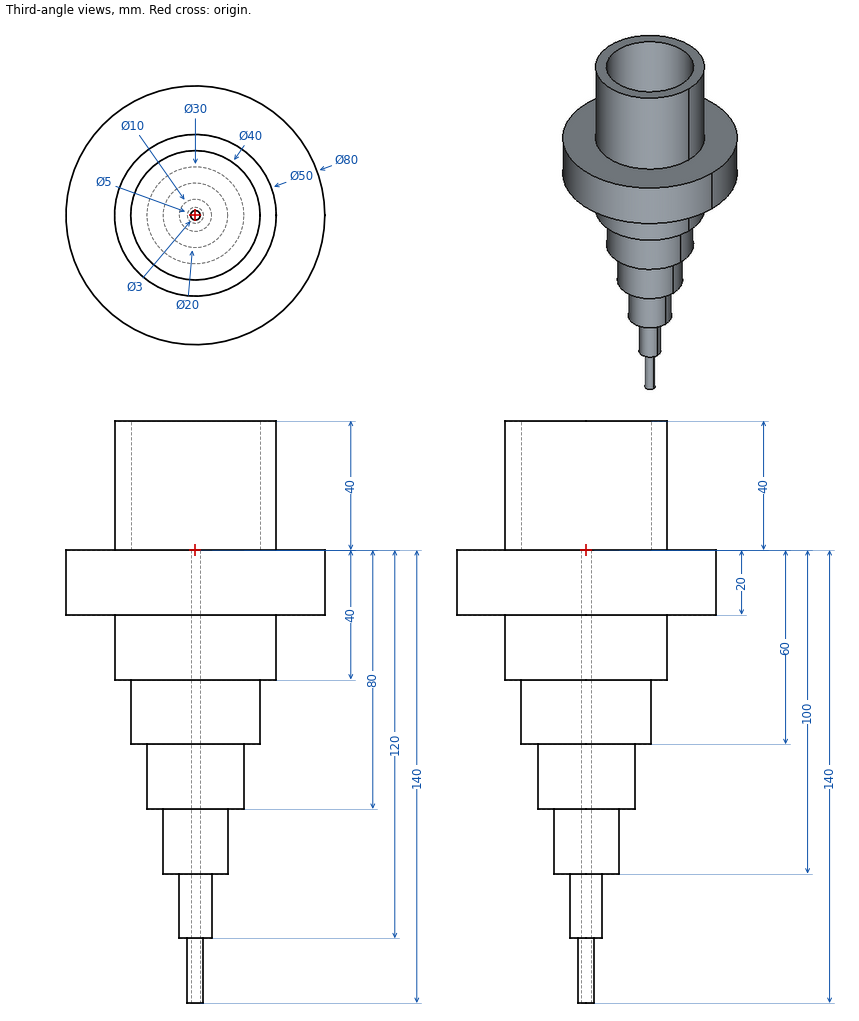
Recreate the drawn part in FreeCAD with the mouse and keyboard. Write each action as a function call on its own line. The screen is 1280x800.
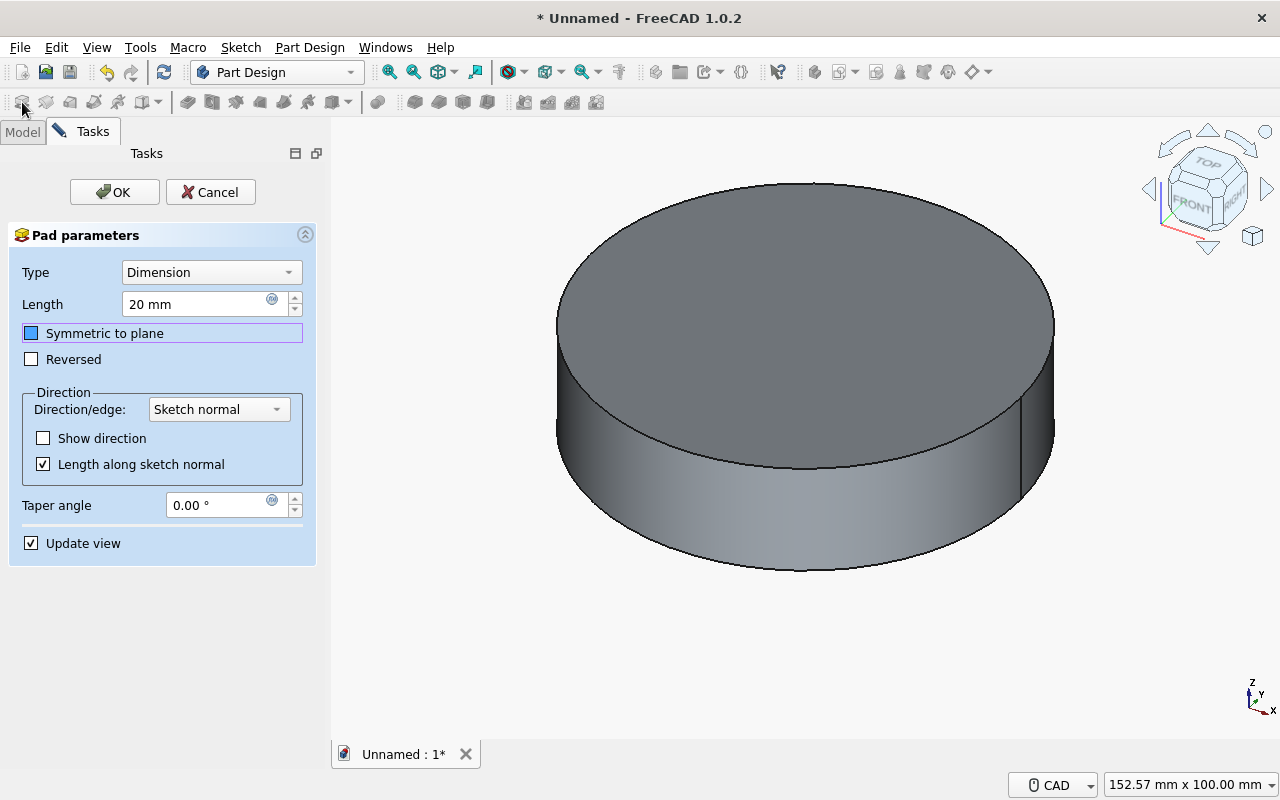
click(30, 359)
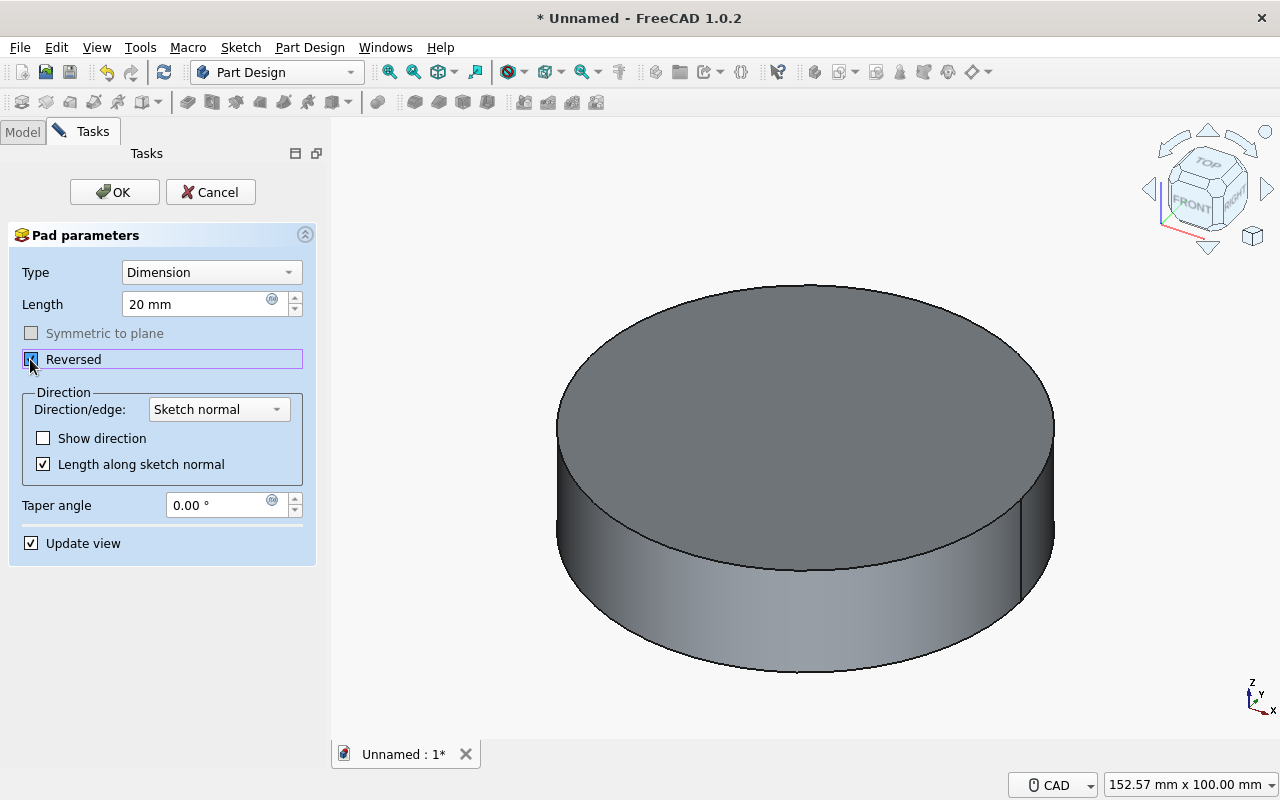
click(115, 192)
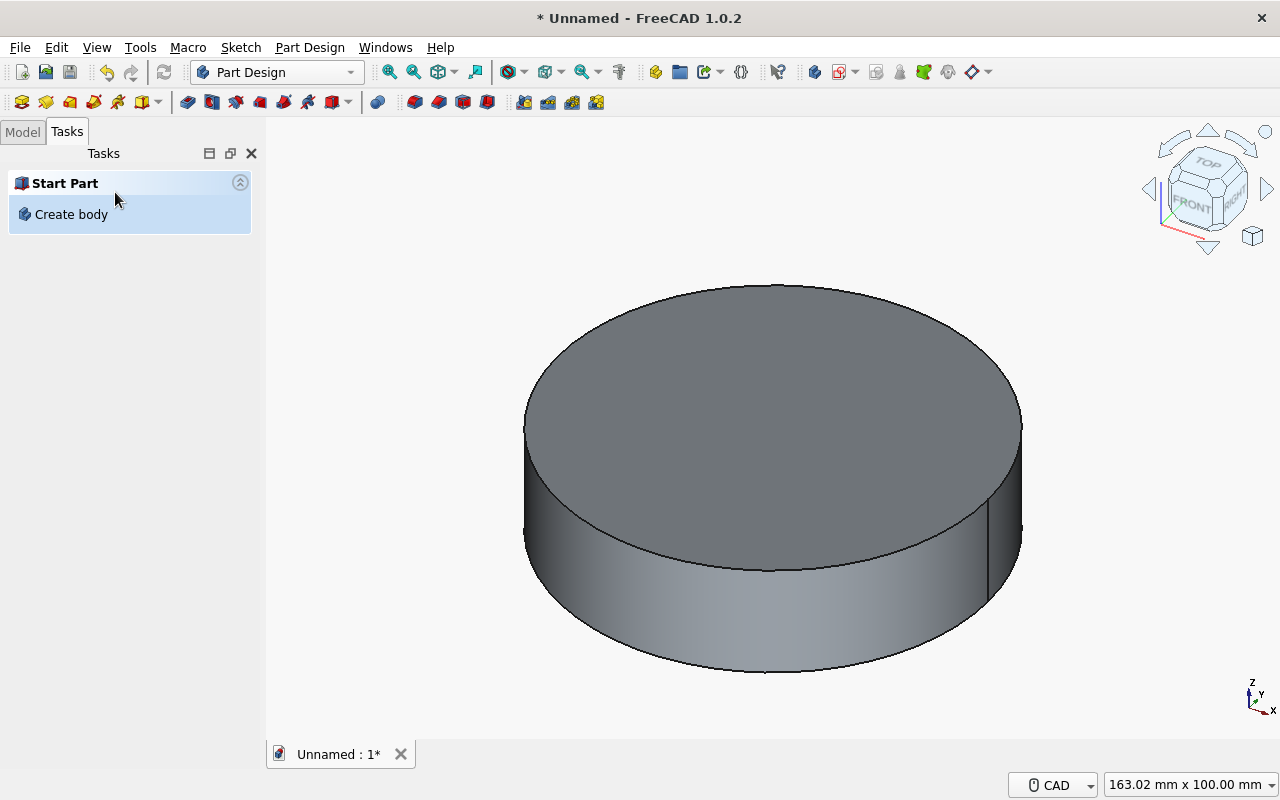
click(840, 72)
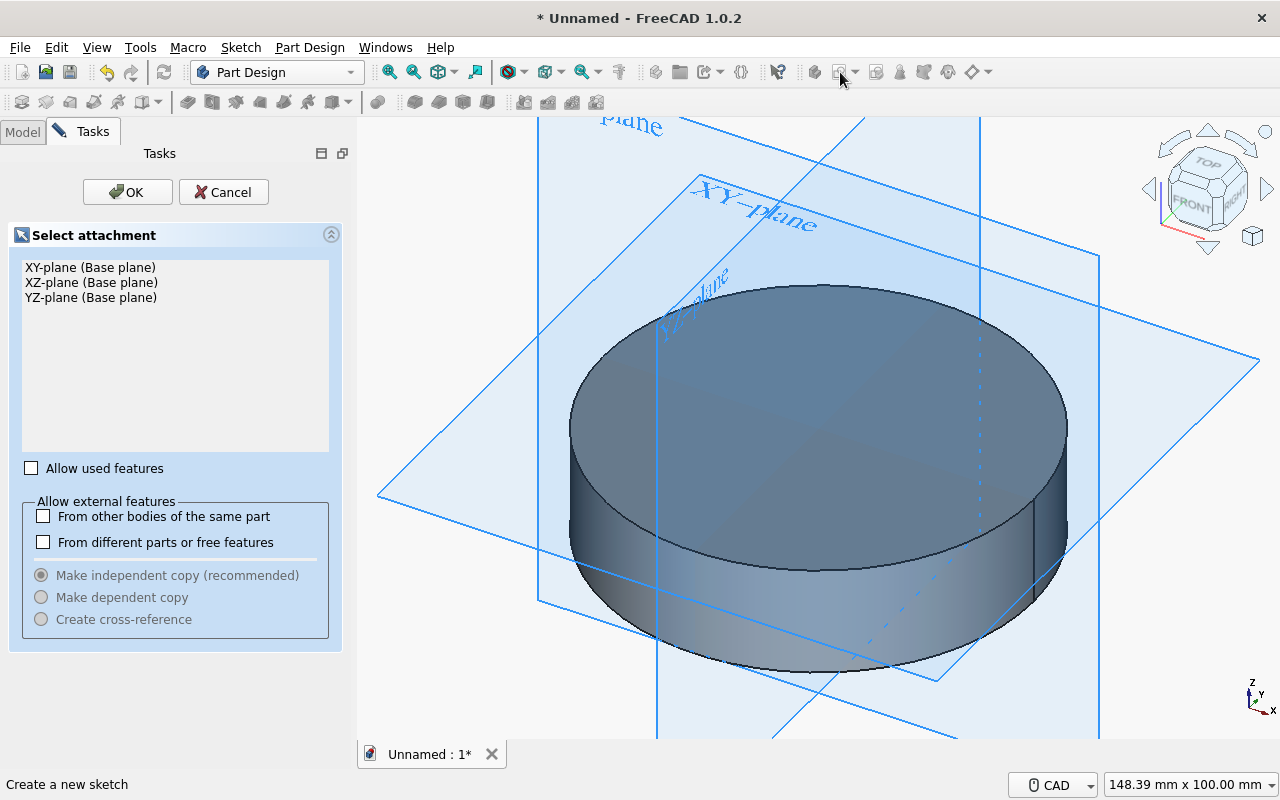
click(82, 268)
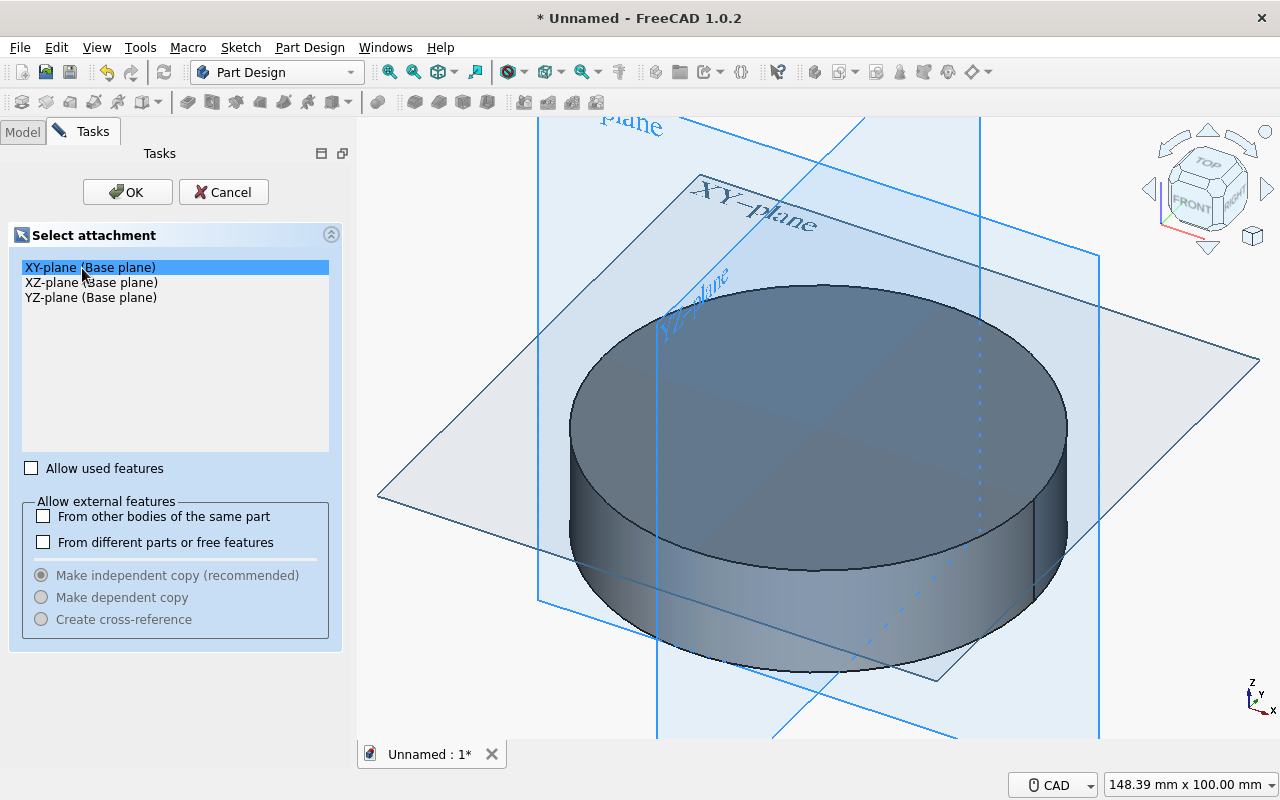
click(128, 192)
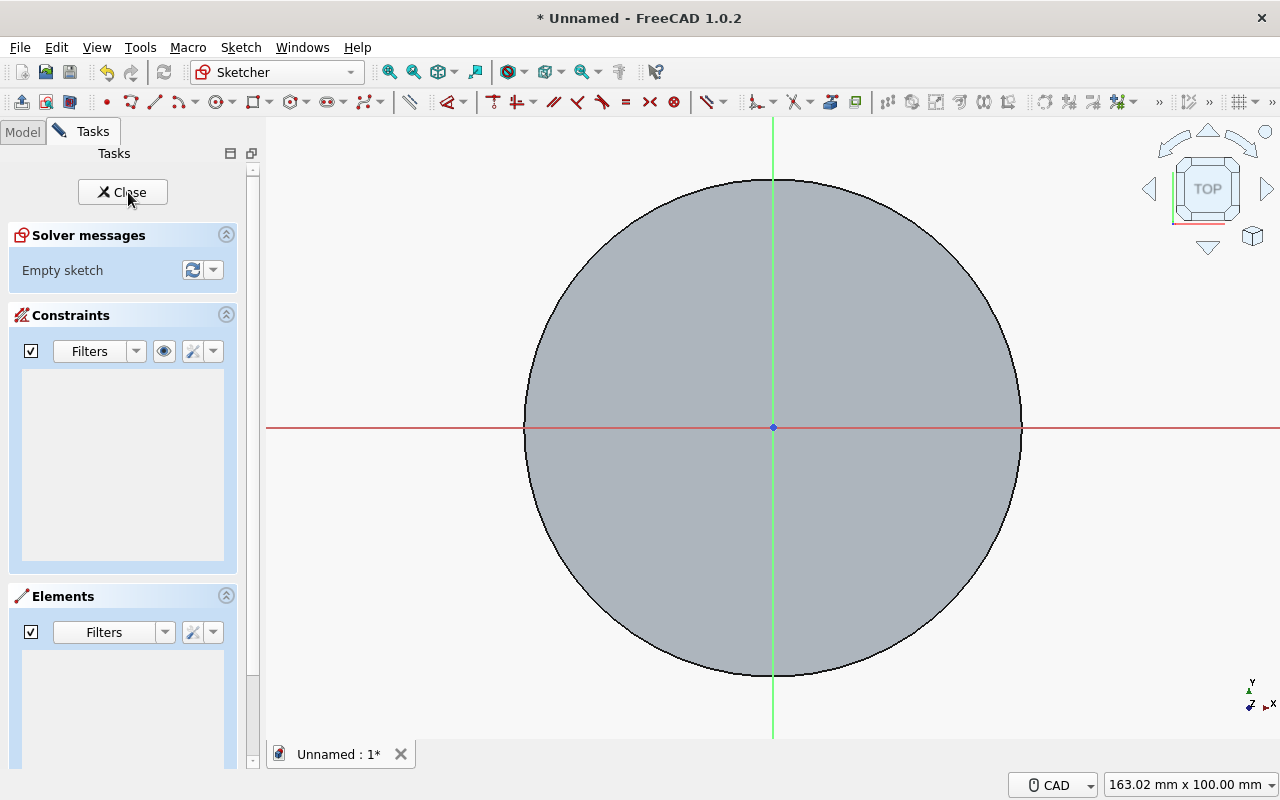
key(g)
key(c)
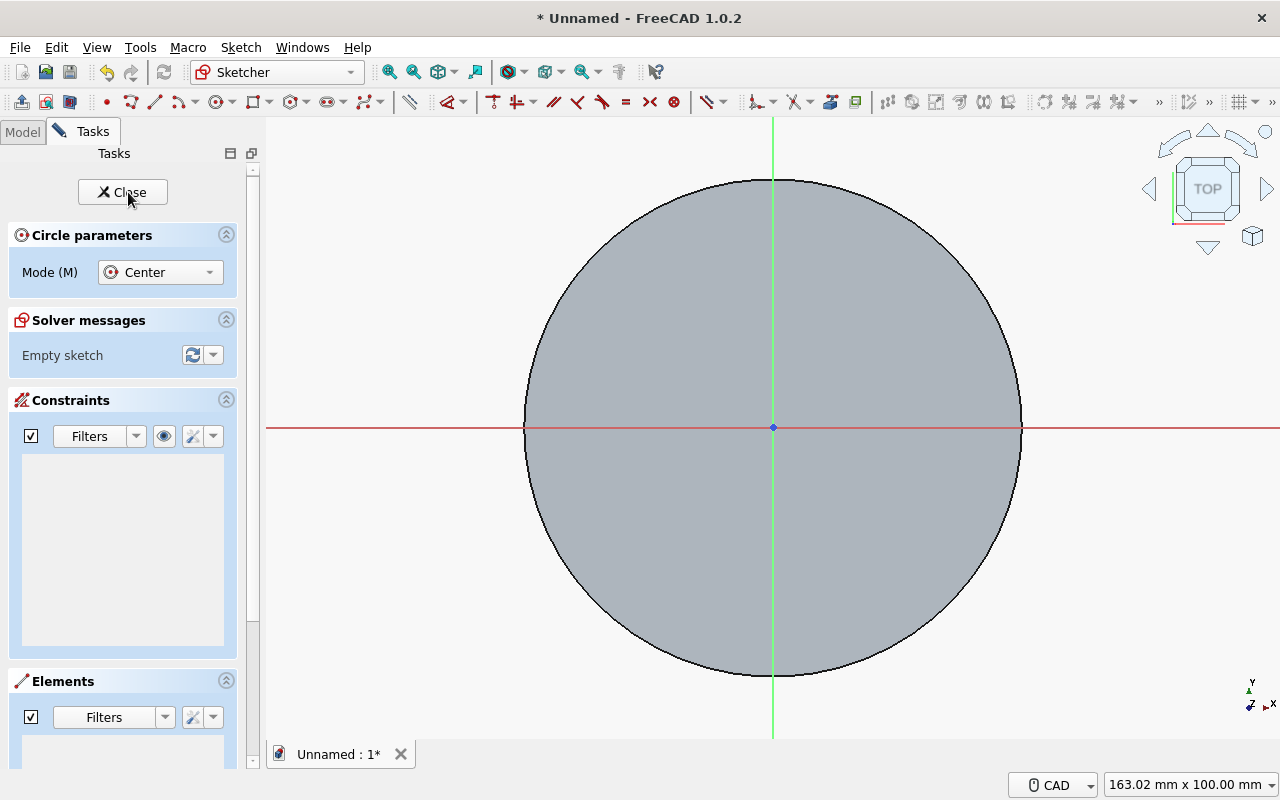
click(773, 428)
move(883, 318)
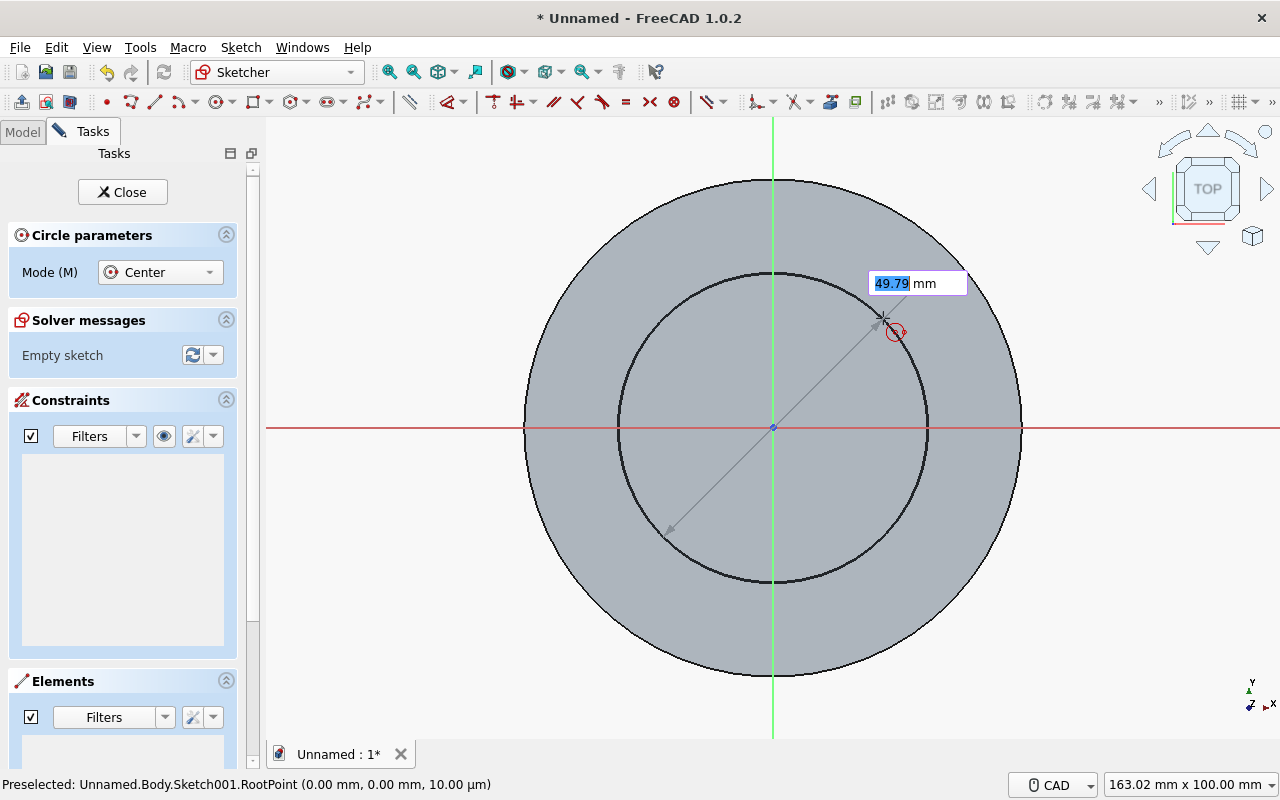
text(50)
key(Return)
key(Escape)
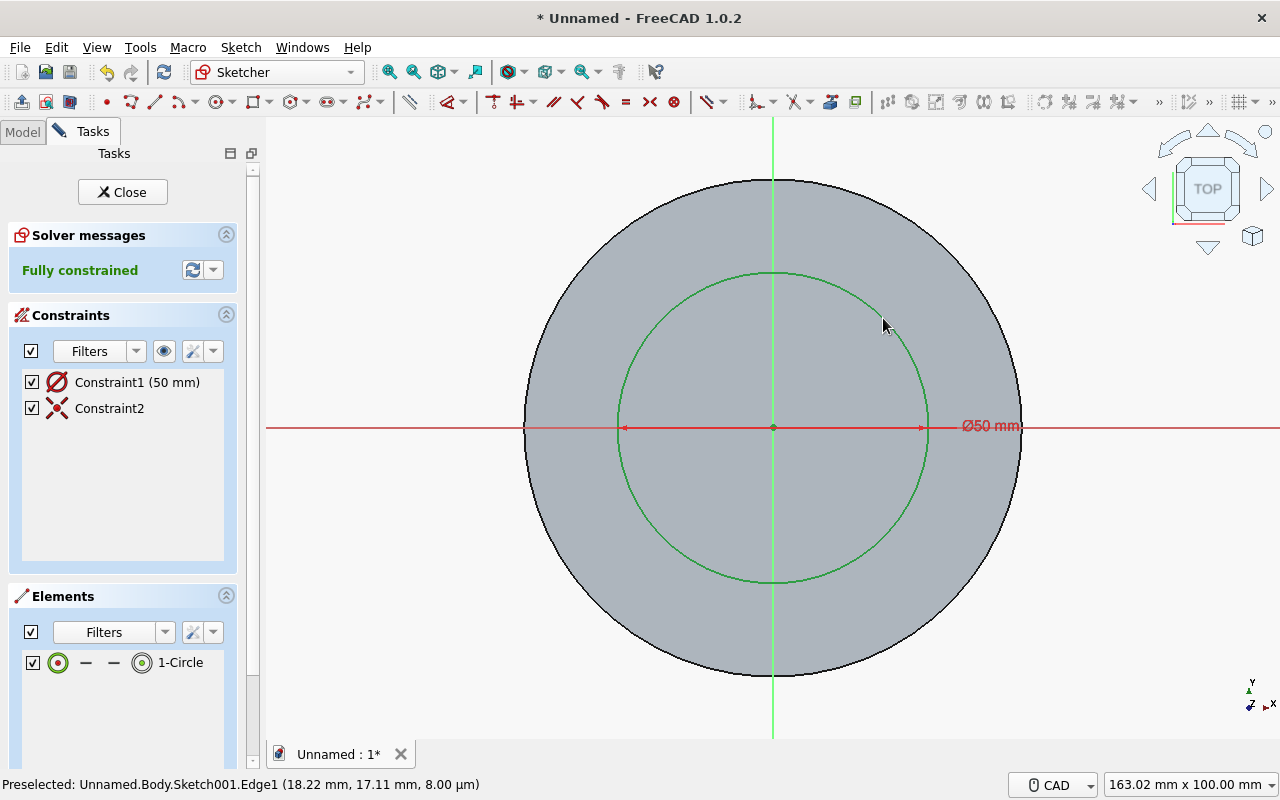
click(123, 192)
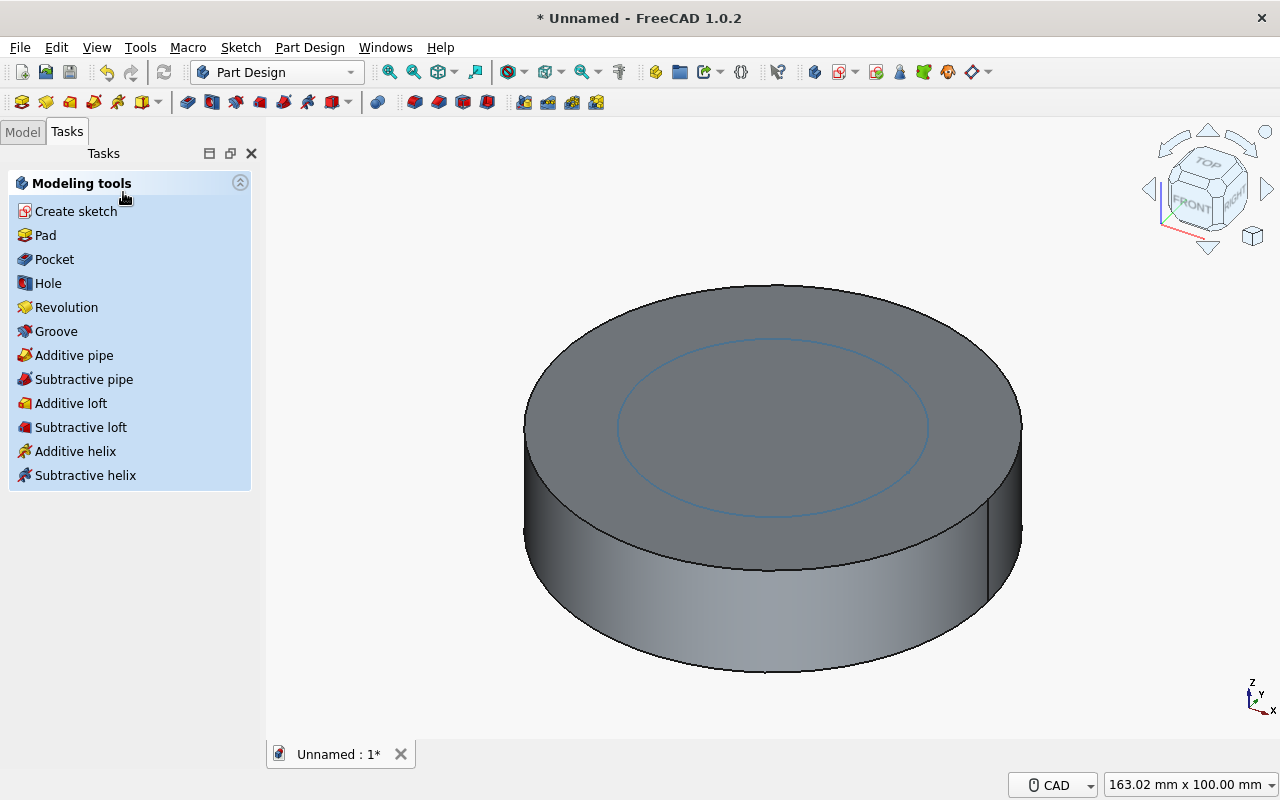
click(22, 102)